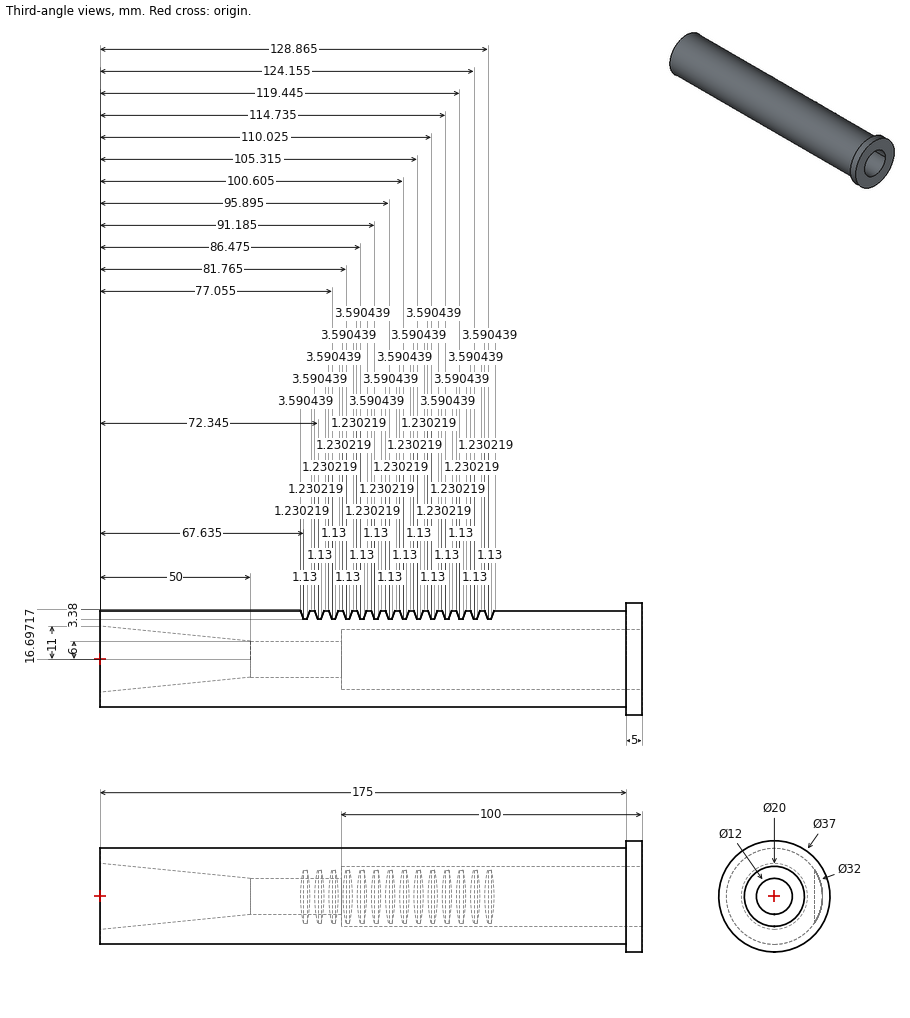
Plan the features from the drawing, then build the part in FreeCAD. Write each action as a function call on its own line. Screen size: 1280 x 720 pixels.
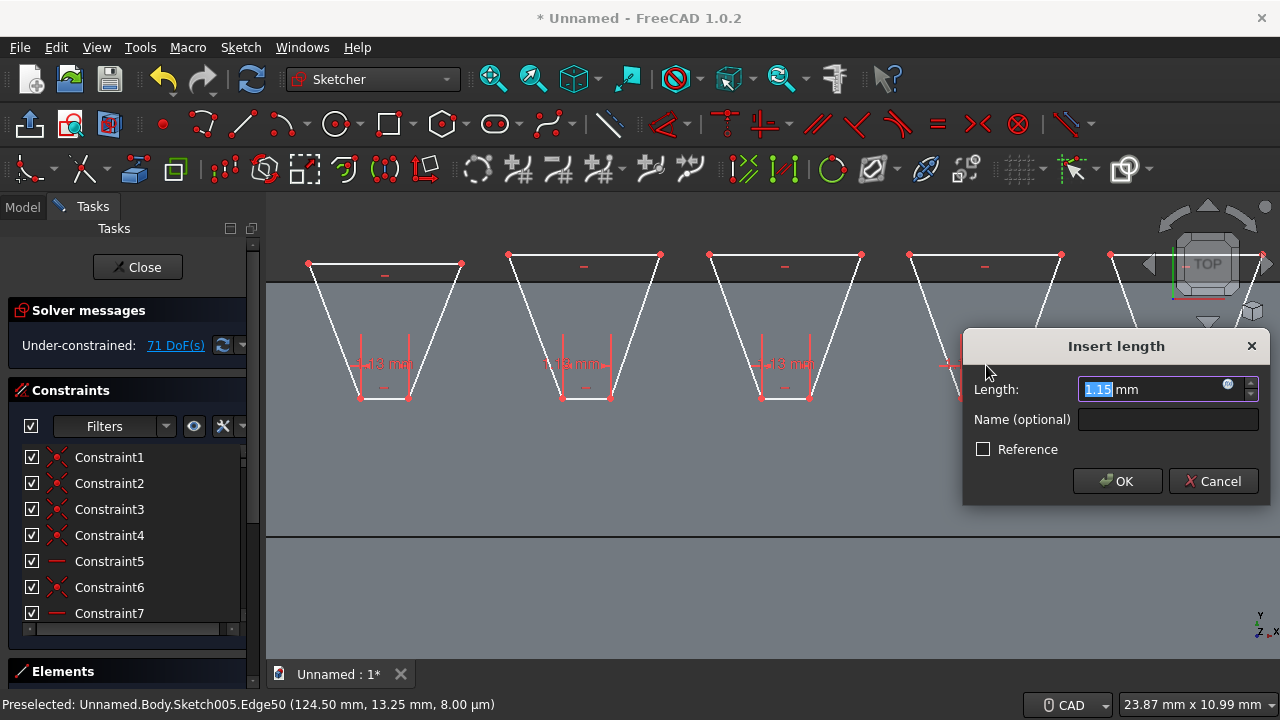
text(1.13)
key(Return)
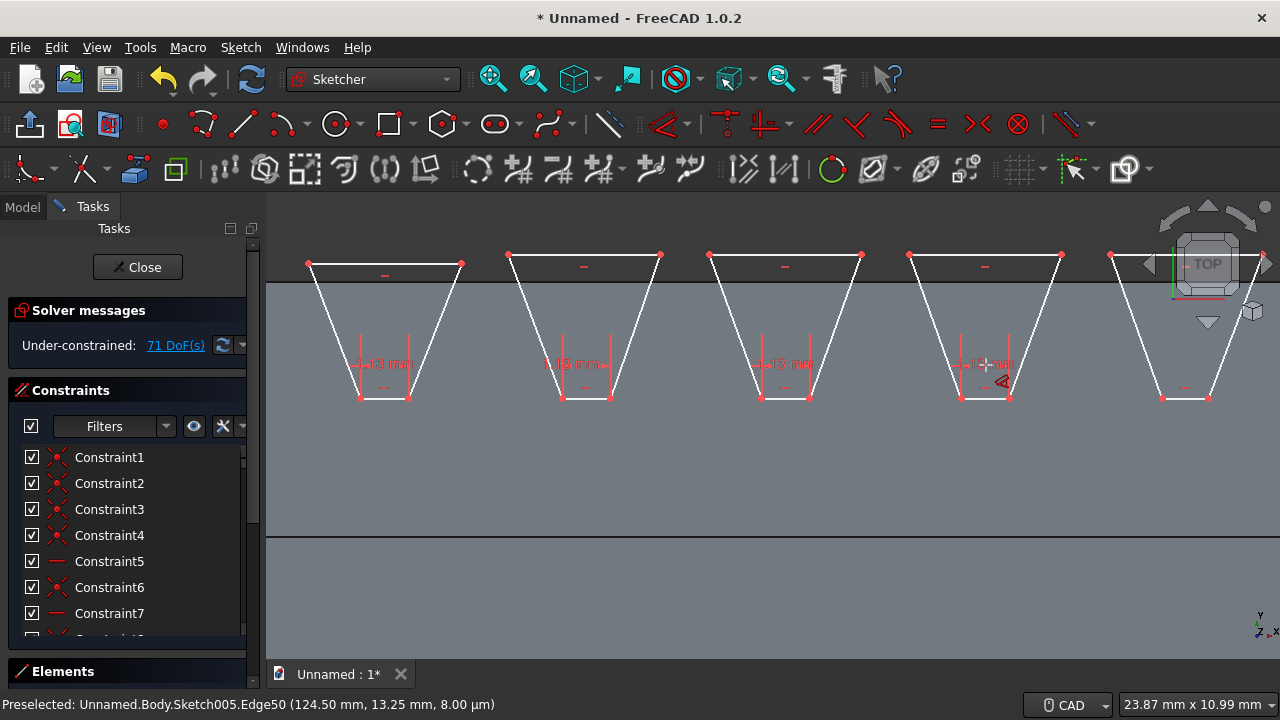
scroll(982, 403, down, 11)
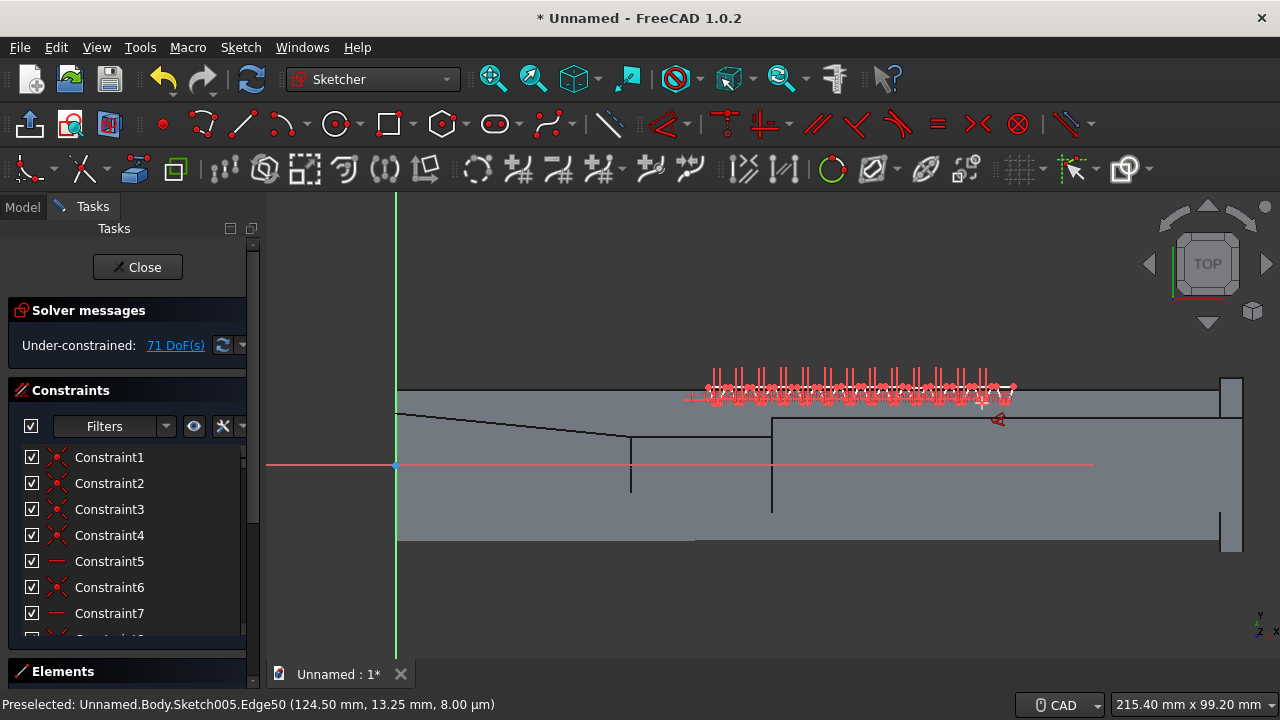
scroll(1004, 403, up, 11)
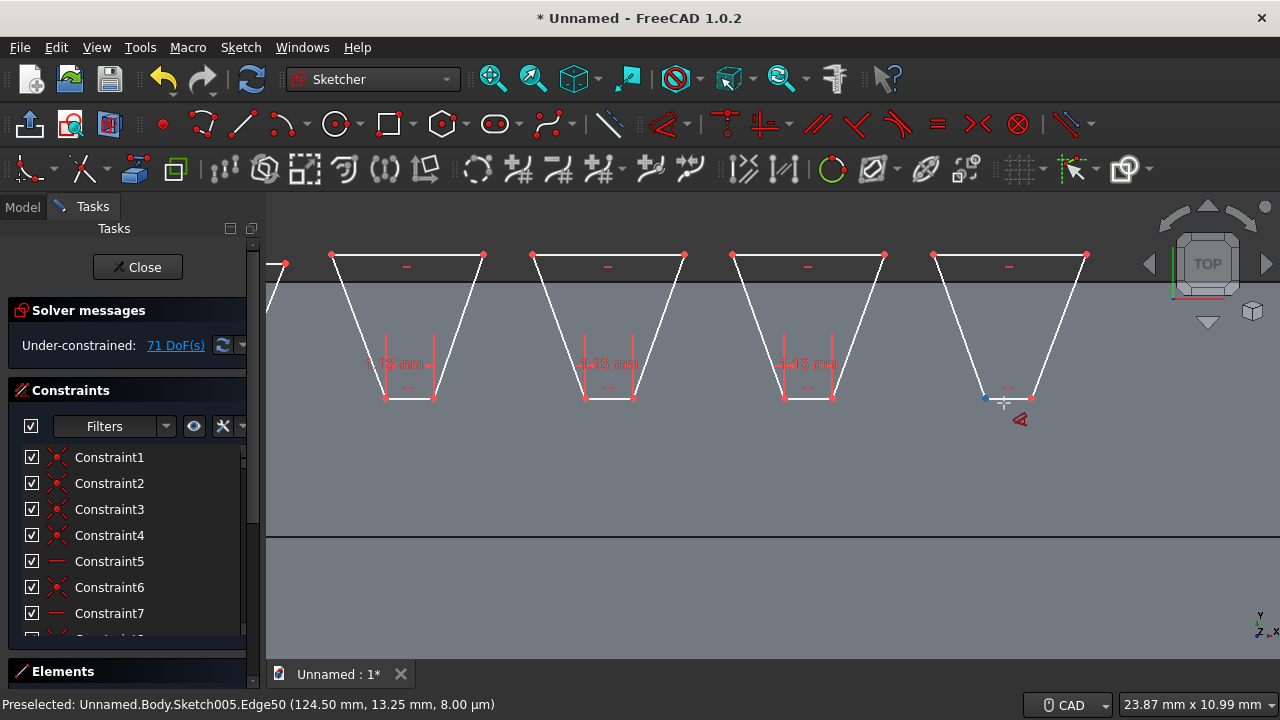
click(999, 399)
click(1009, 365)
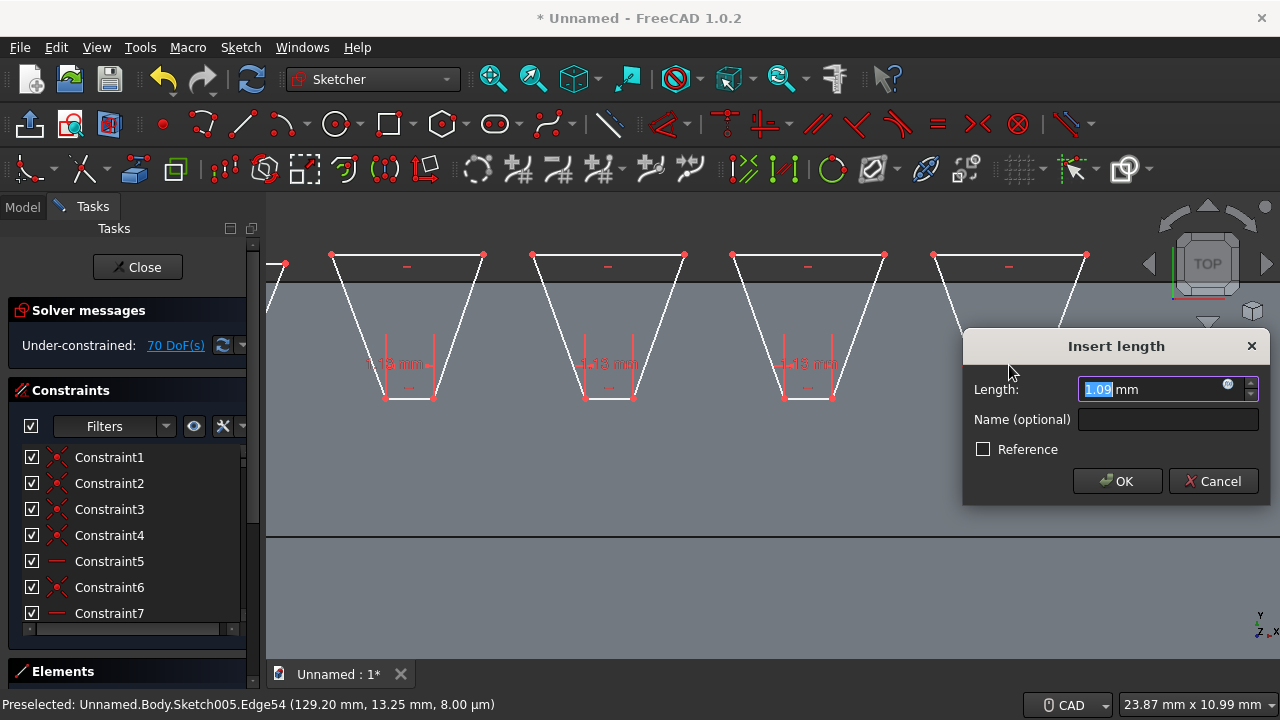
text(1.13)
key(Return)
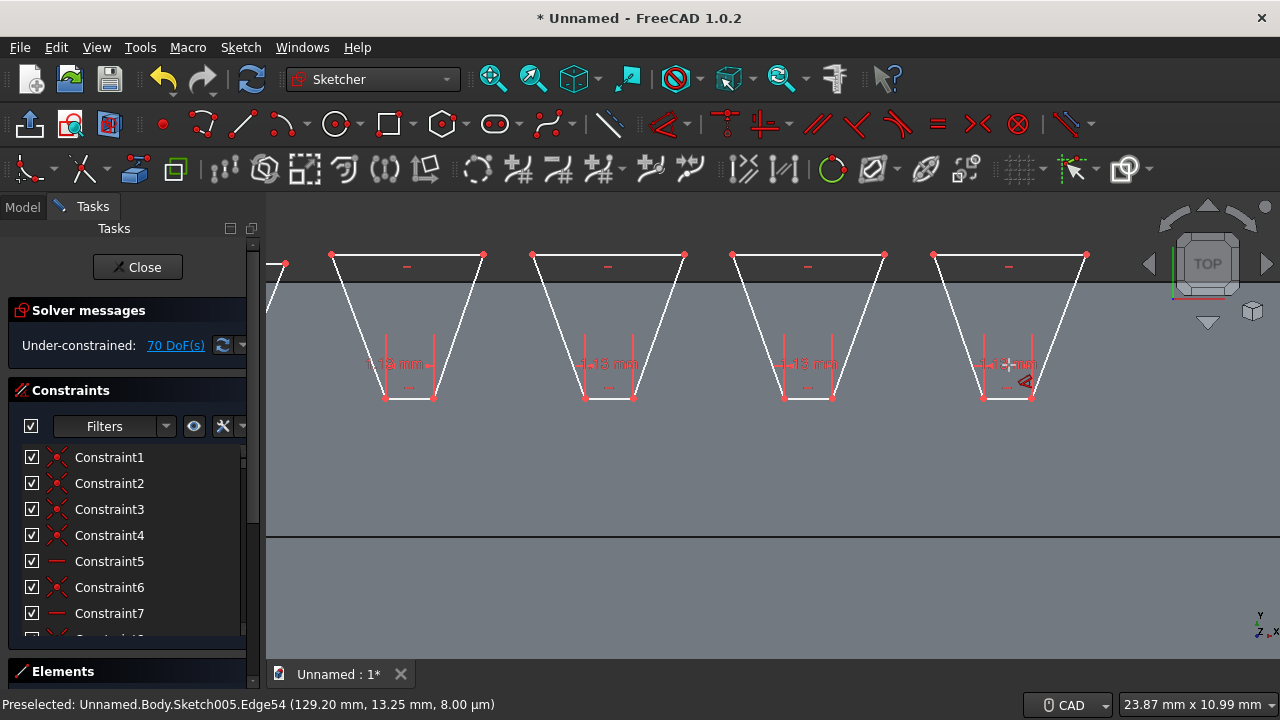
scroll(1004, 403, down, 11)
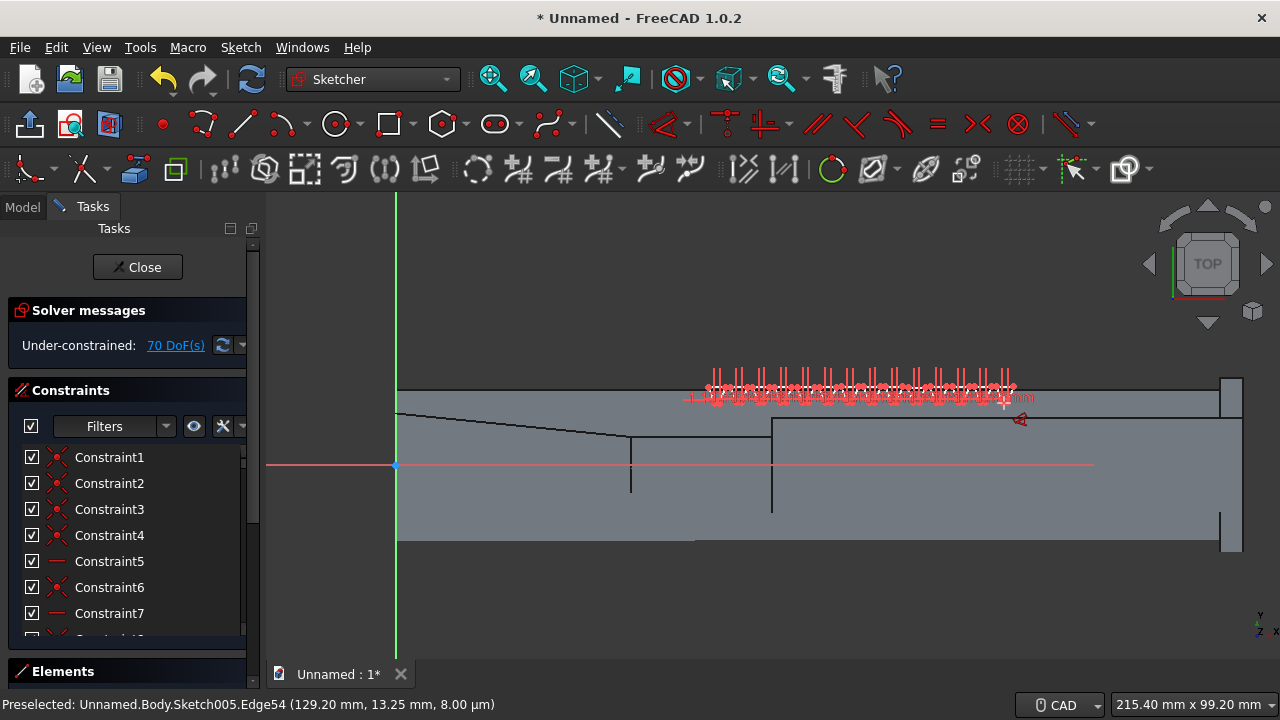
scroll(710, 392, up, 6)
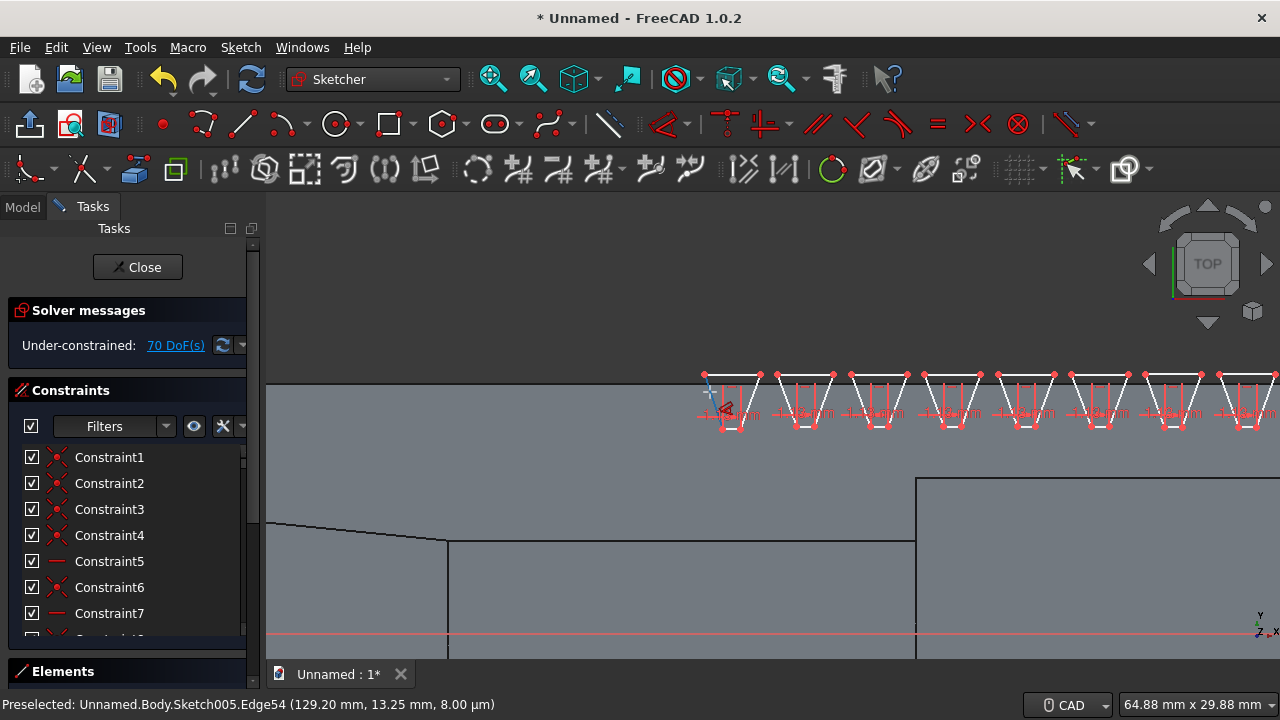
click(710, 391)
click(671, 390)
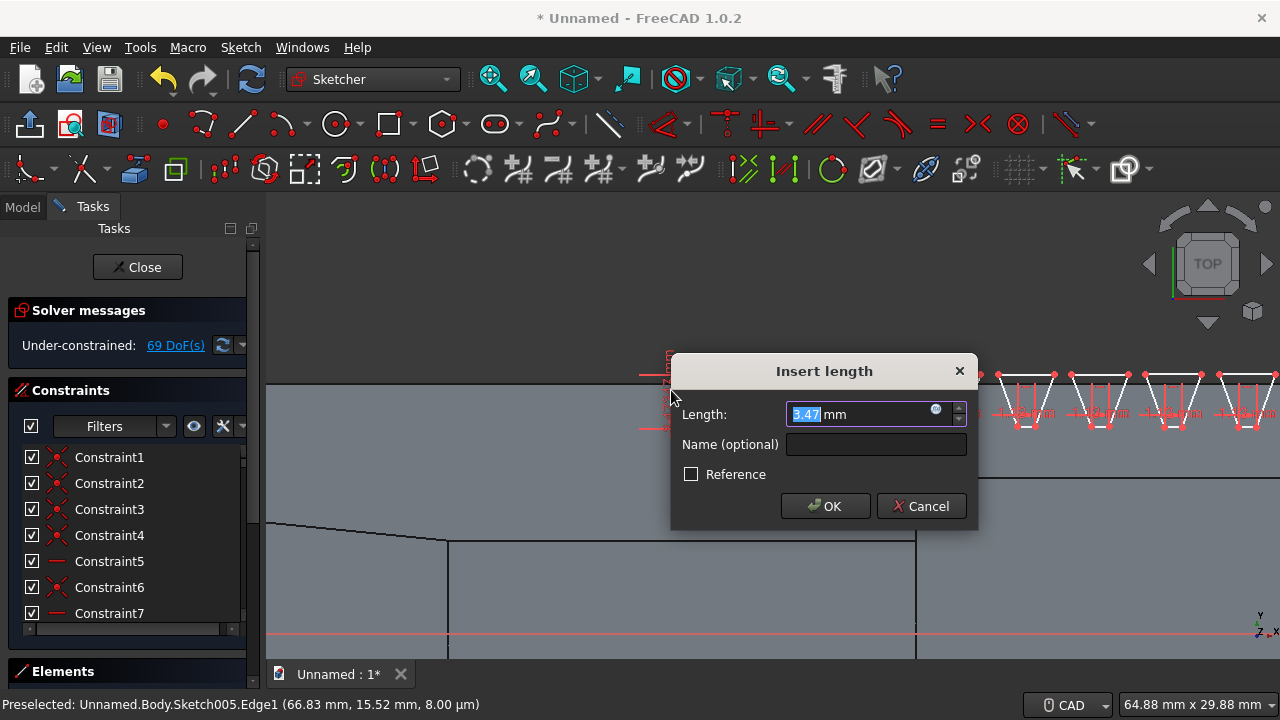
text(3.38)
key(Return)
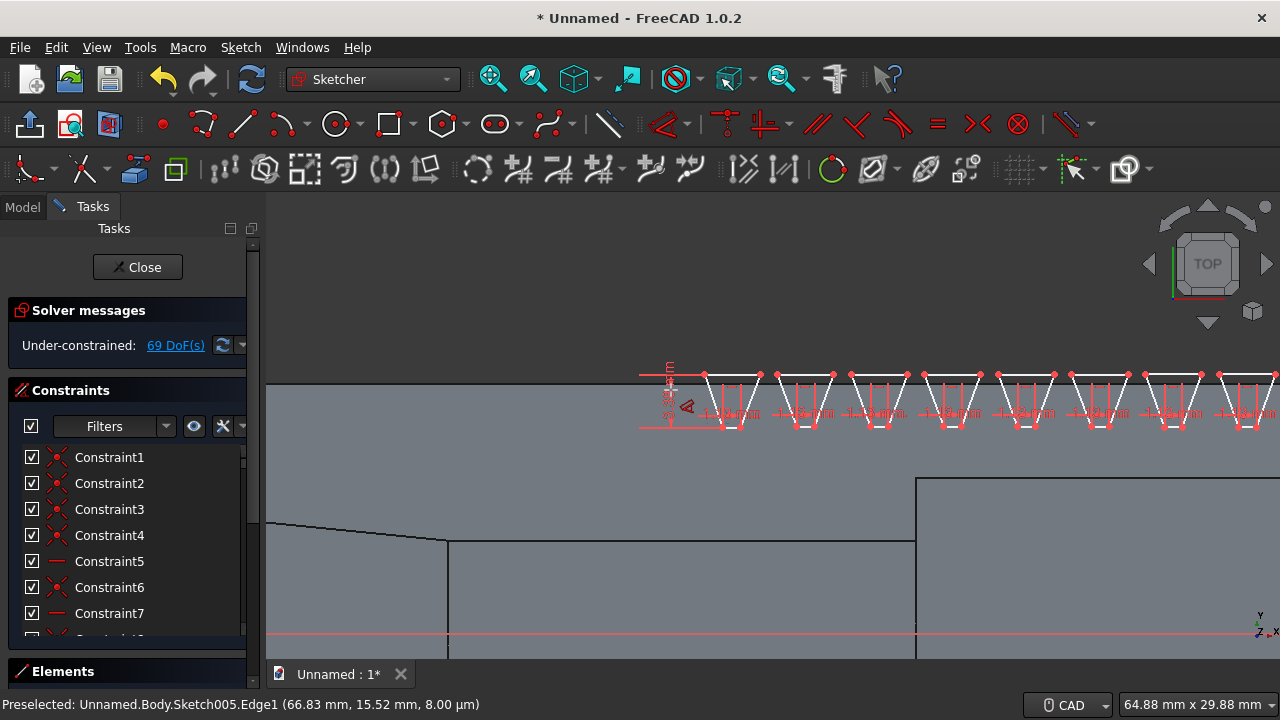
click(783, 391)
click(879, 389)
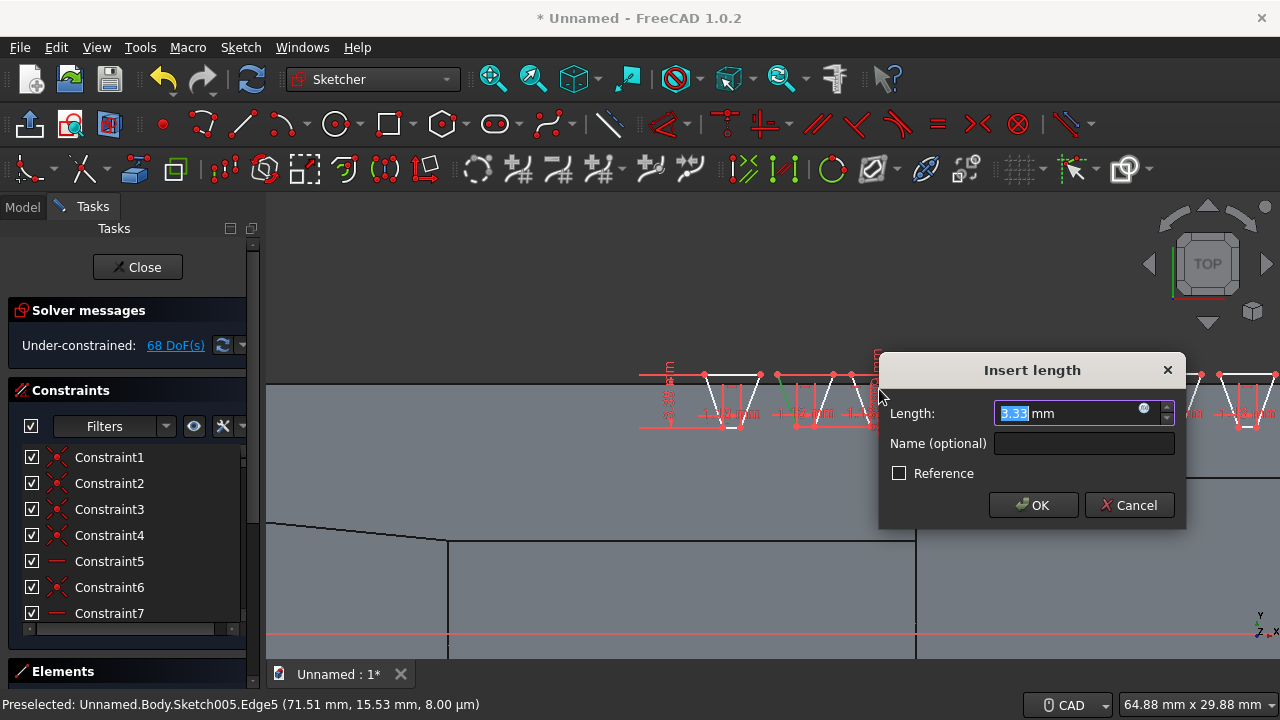
text(3.38)
key(Return)